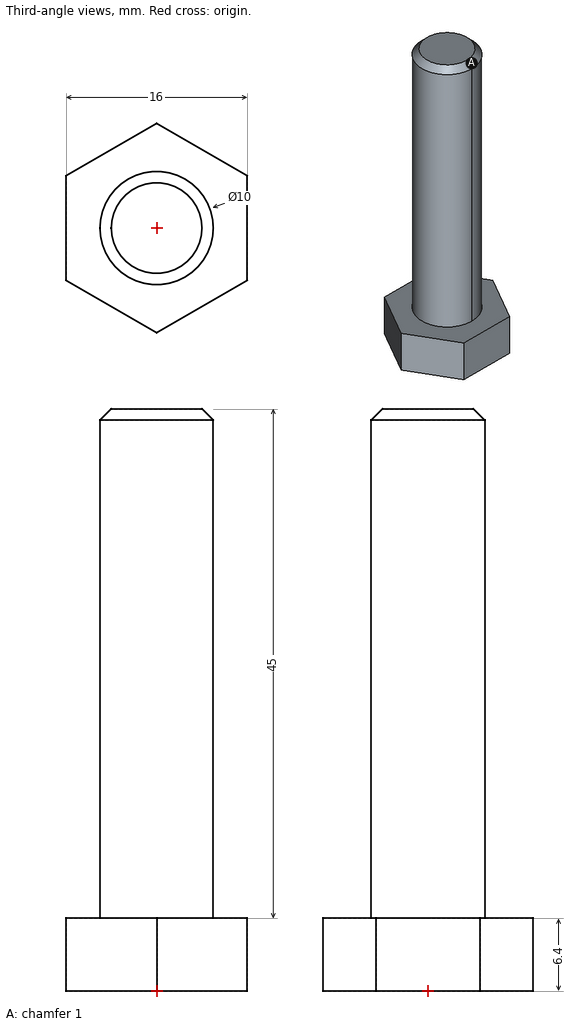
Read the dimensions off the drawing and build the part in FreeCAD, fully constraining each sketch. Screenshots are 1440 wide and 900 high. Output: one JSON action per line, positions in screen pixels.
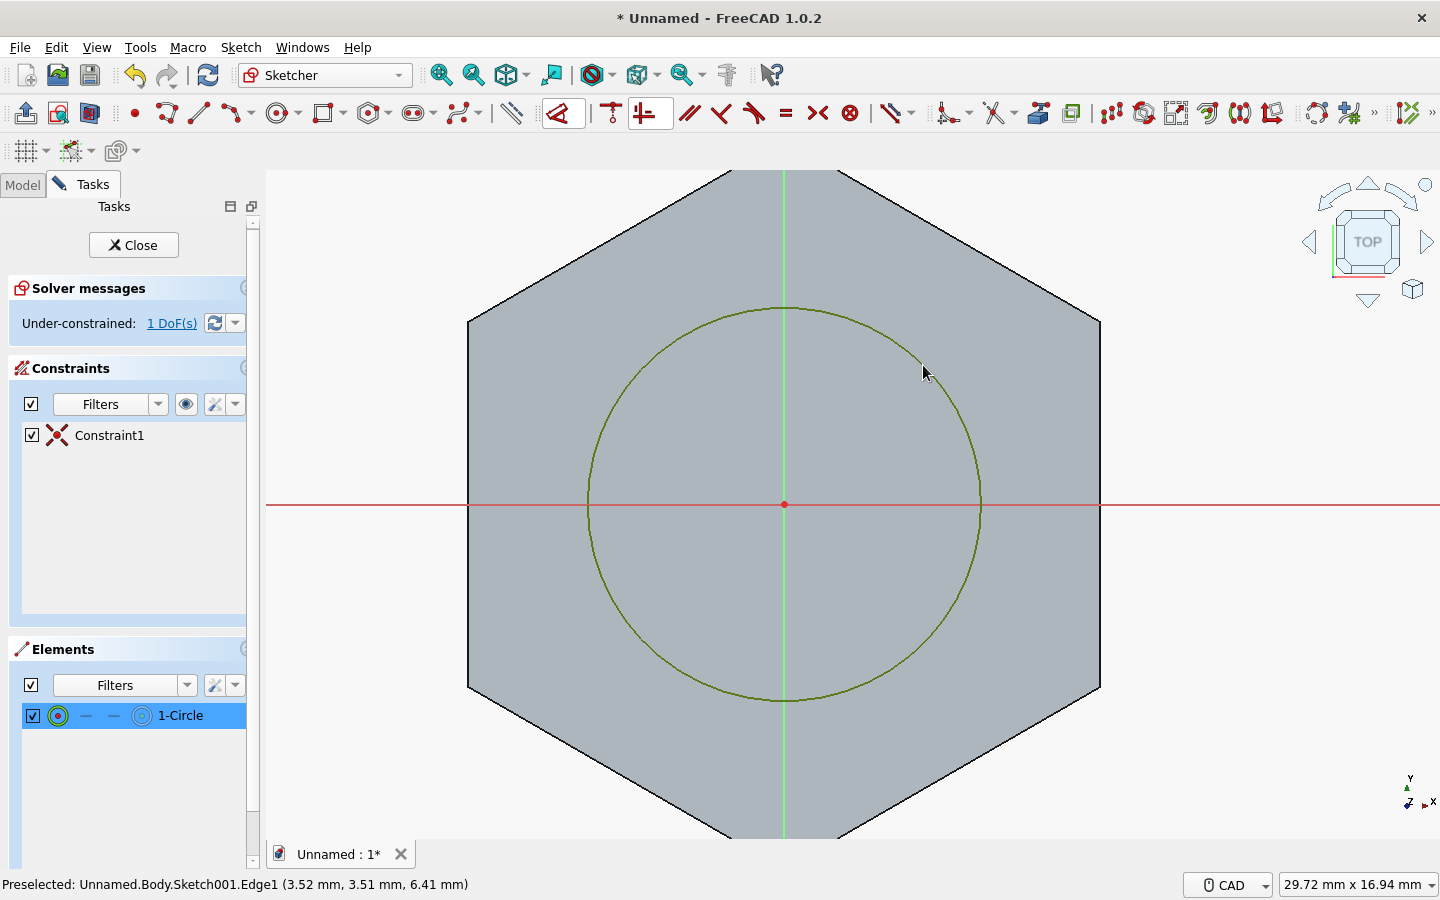
{"action": "key", "text": "k o"}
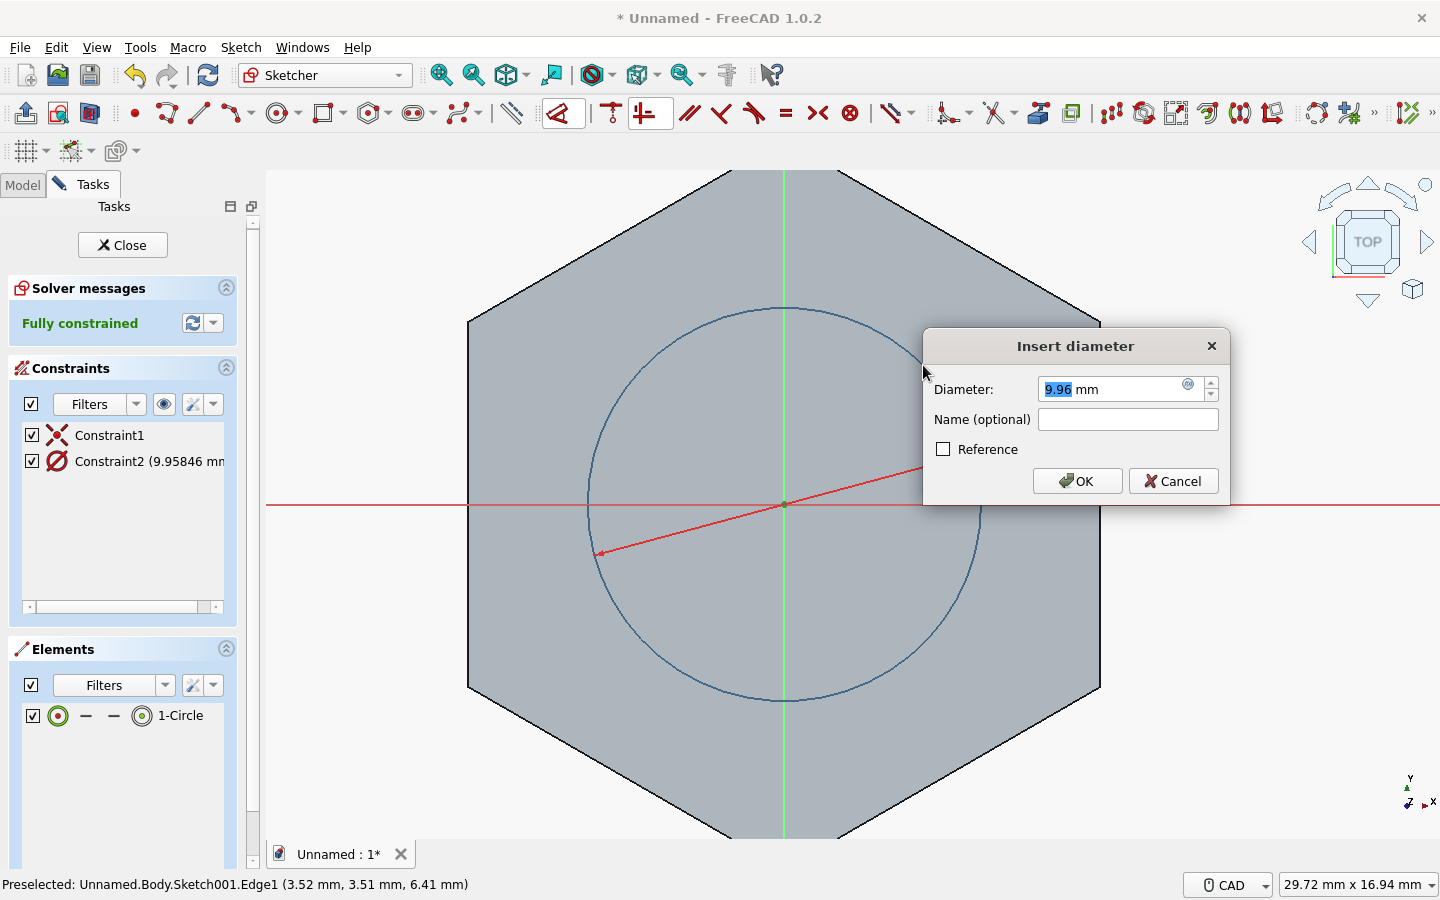
{"action": "type", "text": "10"}
{"action": "key", "text": "Return"}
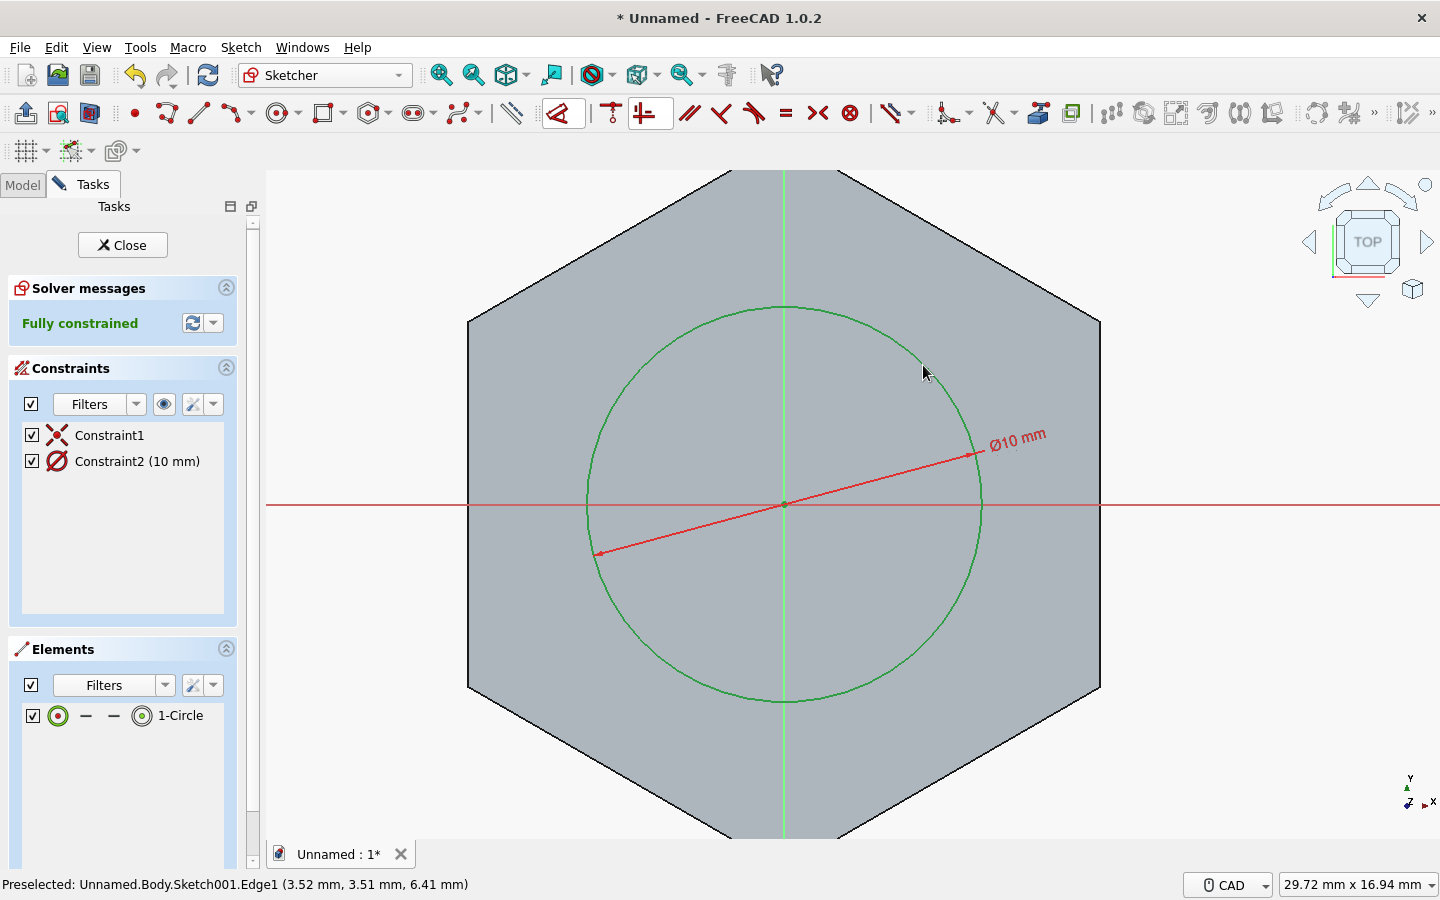
{"action": "left_click", "coordinate": [123, 245]}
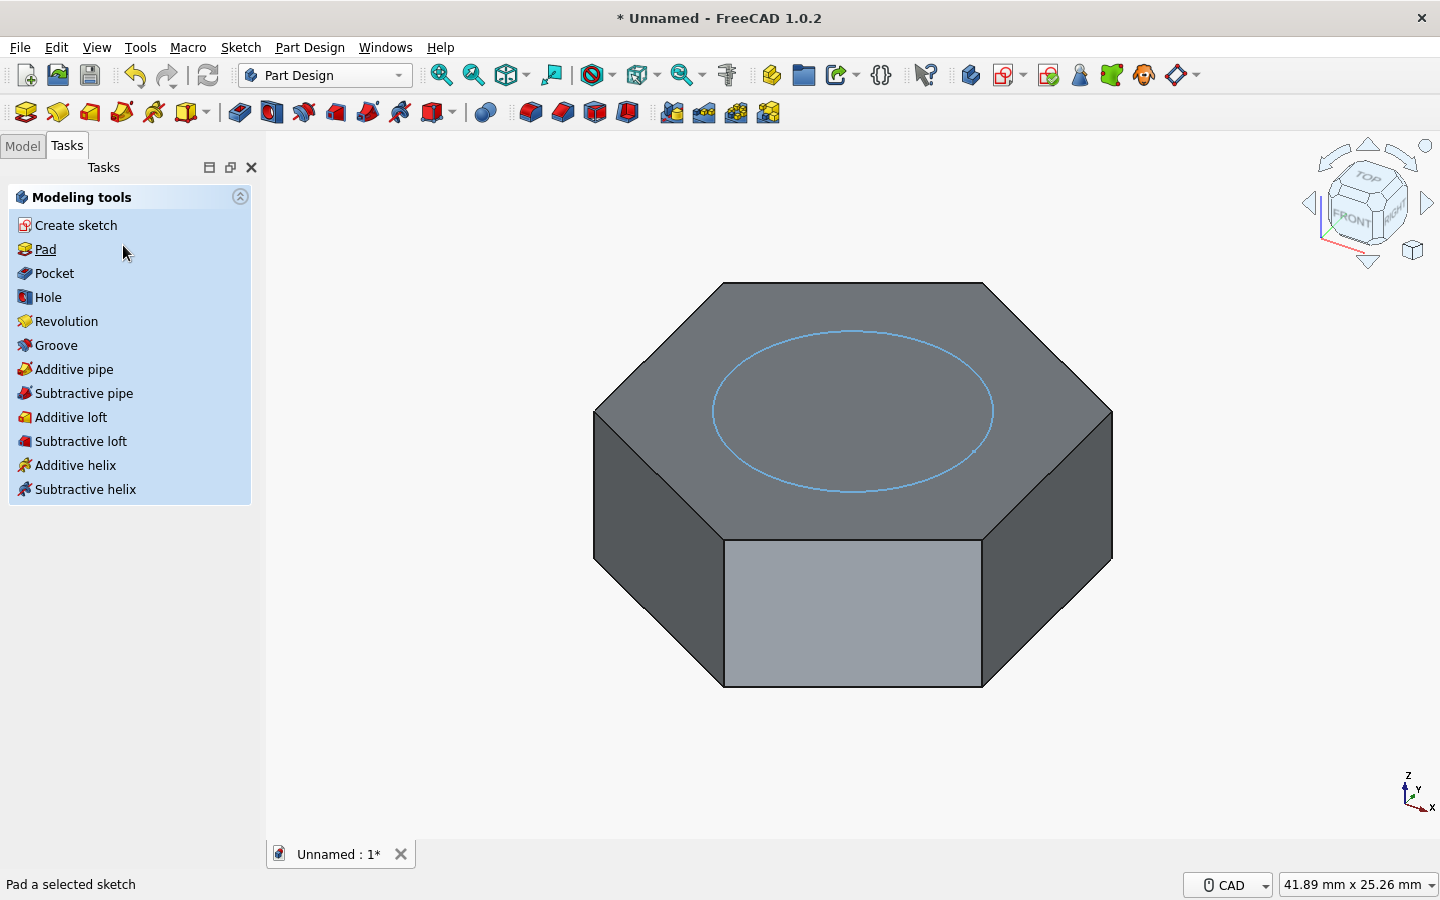
{"action": "left_click", "coordinate": [26, 112]}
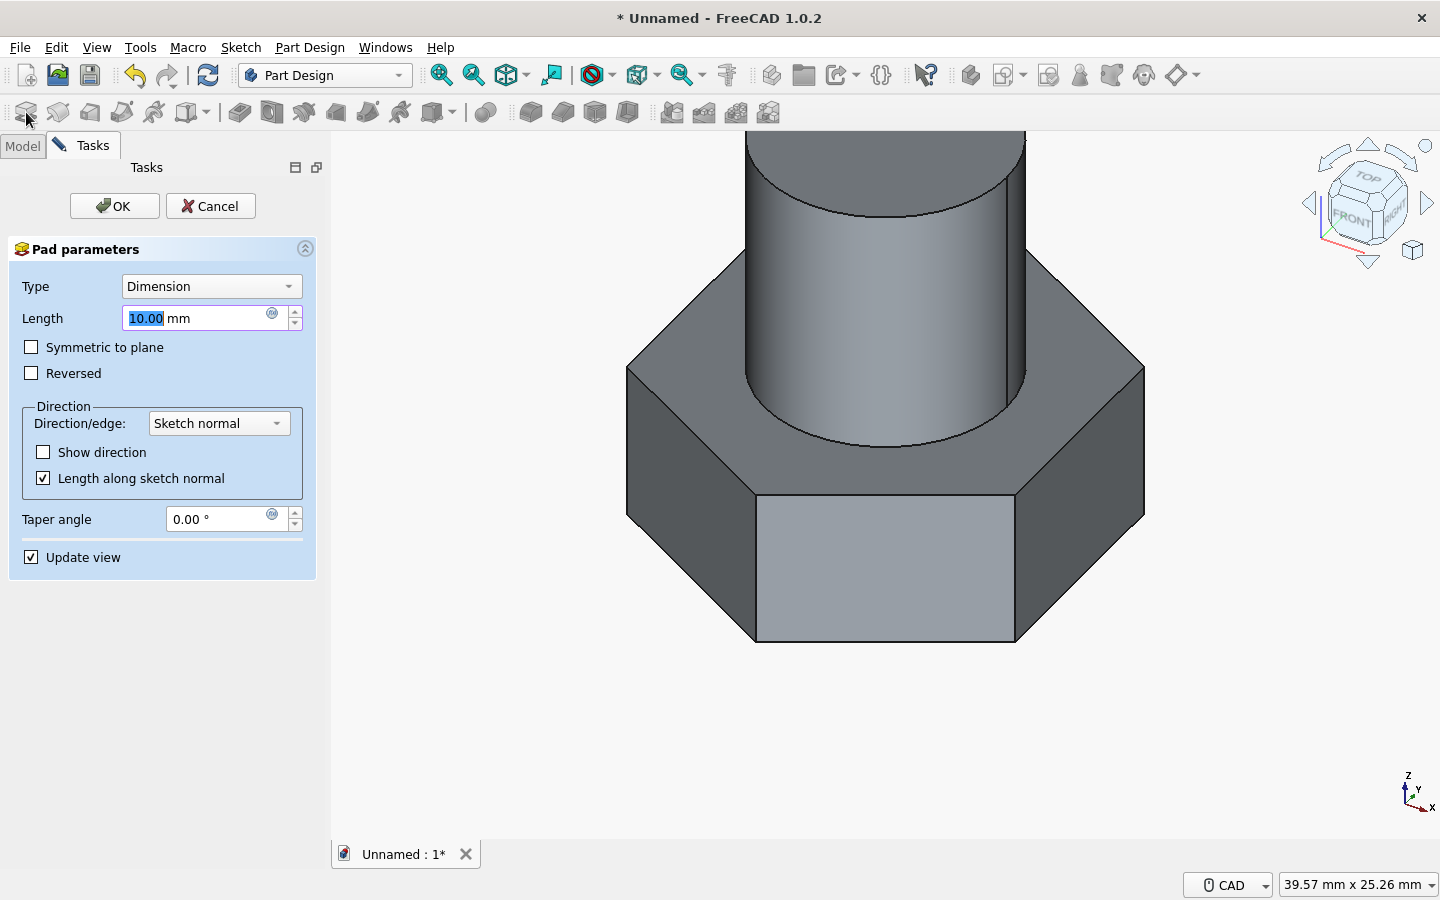
{"action": "type", "text": "45"}
{"action": "key", "text": "Tab"}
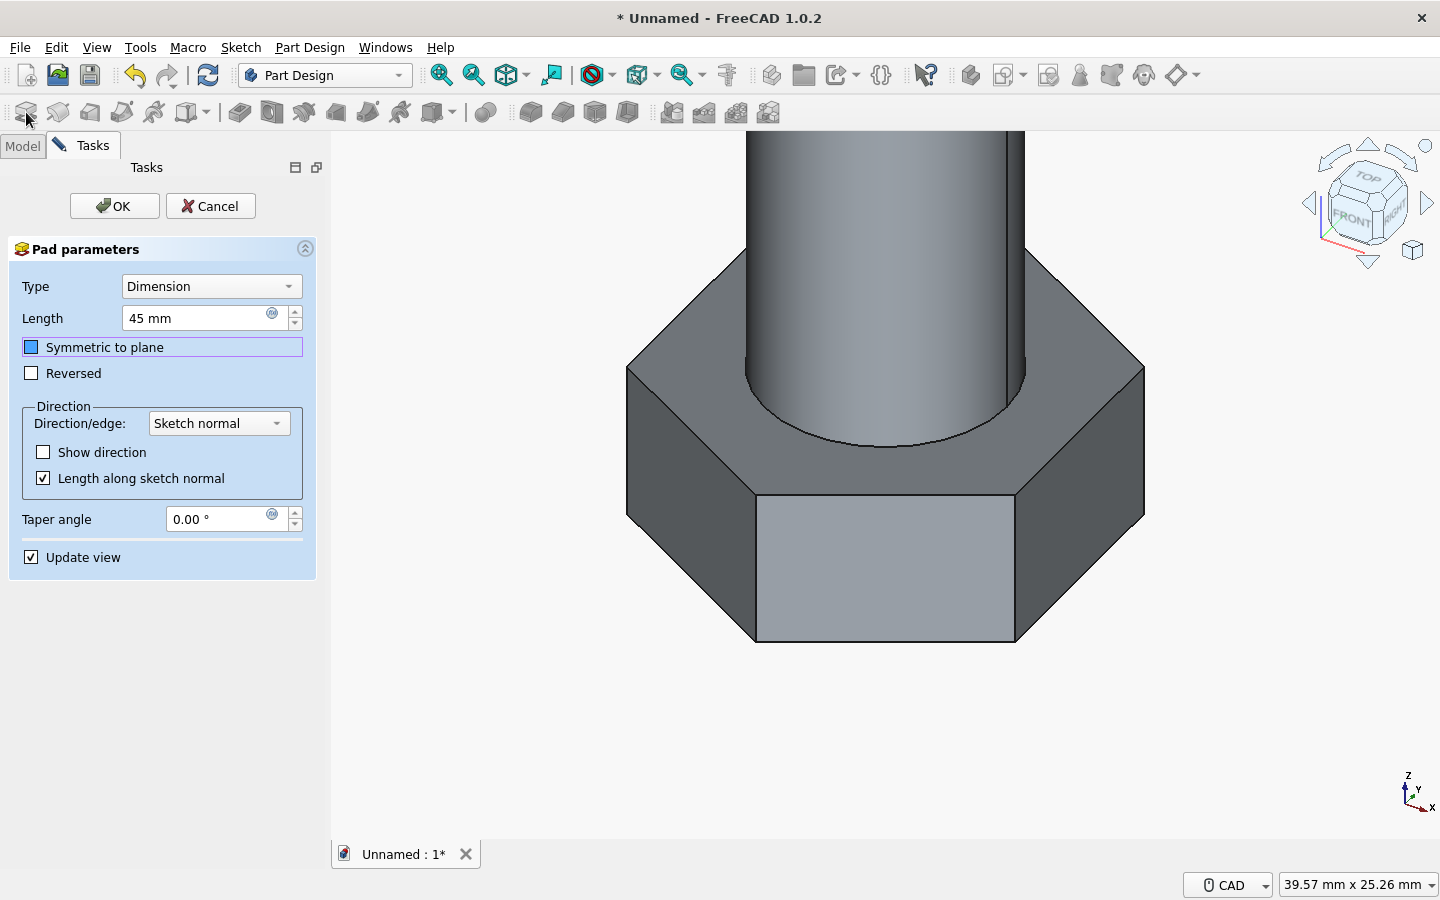
{"action": "left_click", "coordinate": [115, 206]}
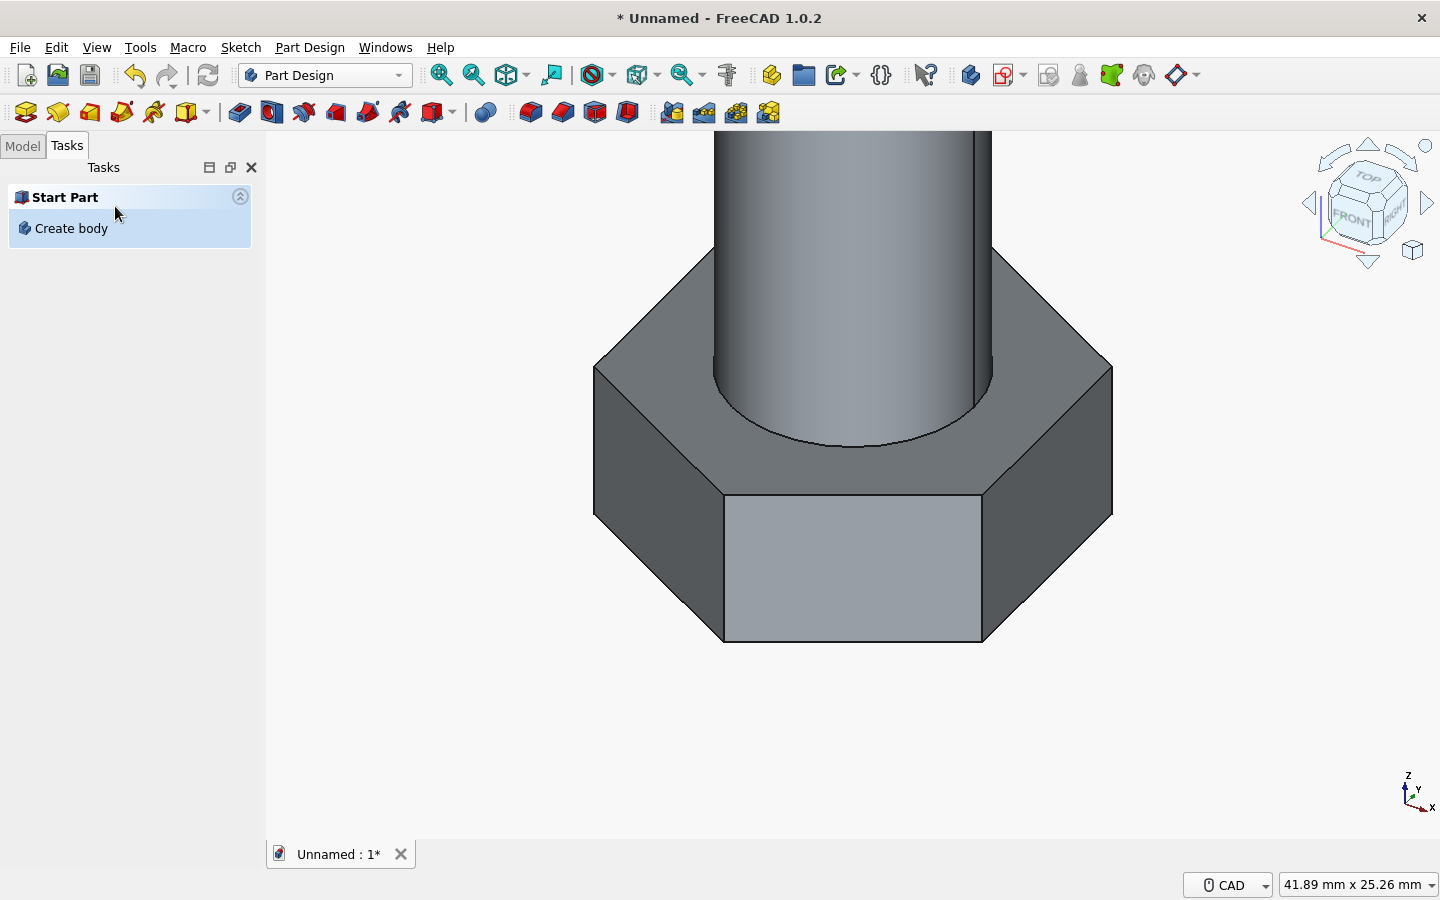
{"action": "left_click", "coordinate": [442, 76]}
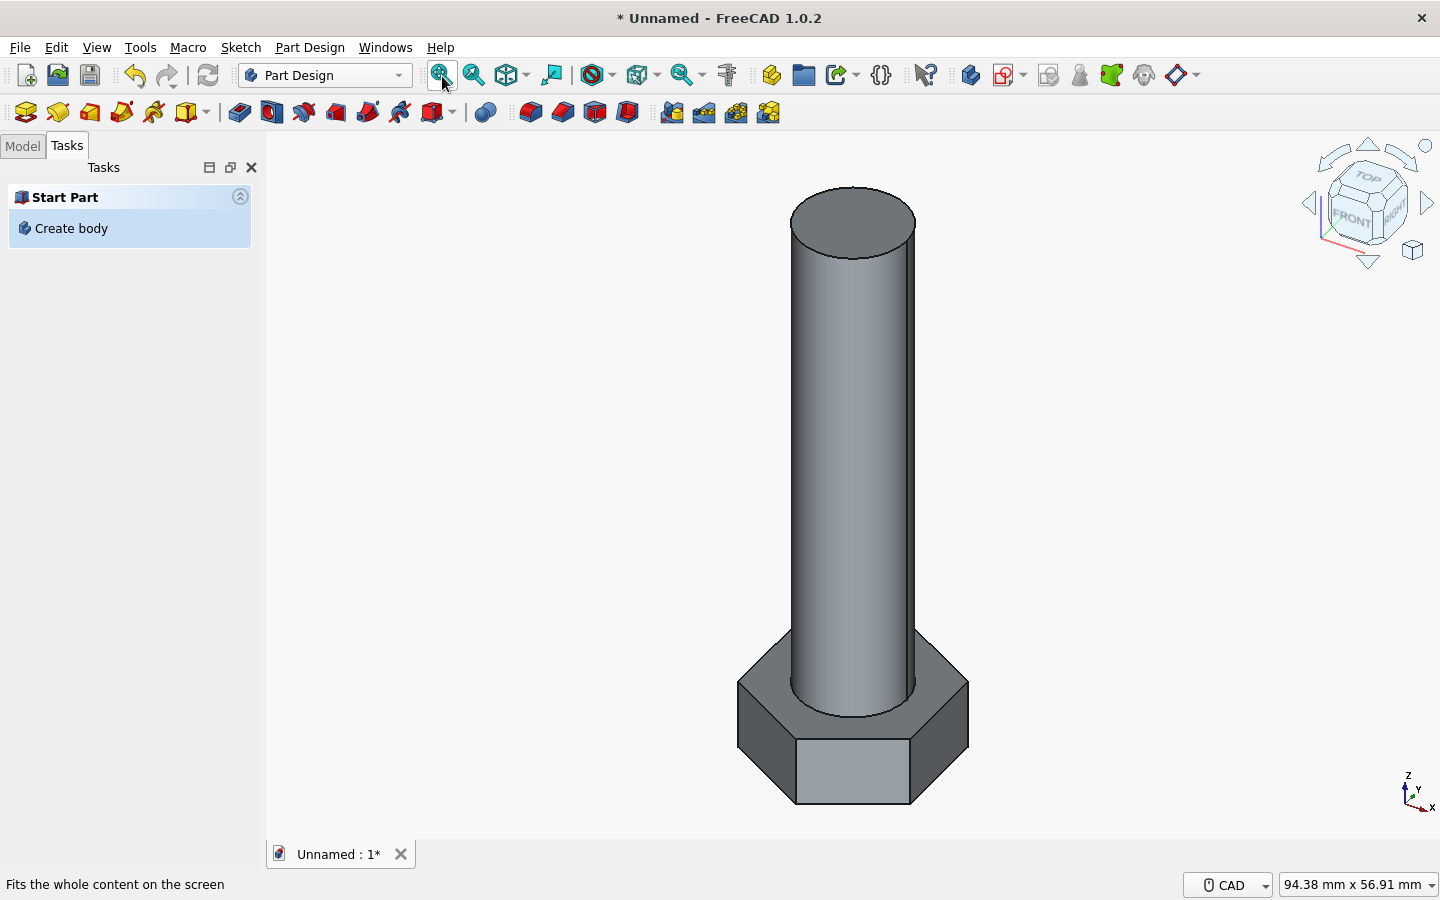
{"action": "left_click", "coordinate": [791, 226]}